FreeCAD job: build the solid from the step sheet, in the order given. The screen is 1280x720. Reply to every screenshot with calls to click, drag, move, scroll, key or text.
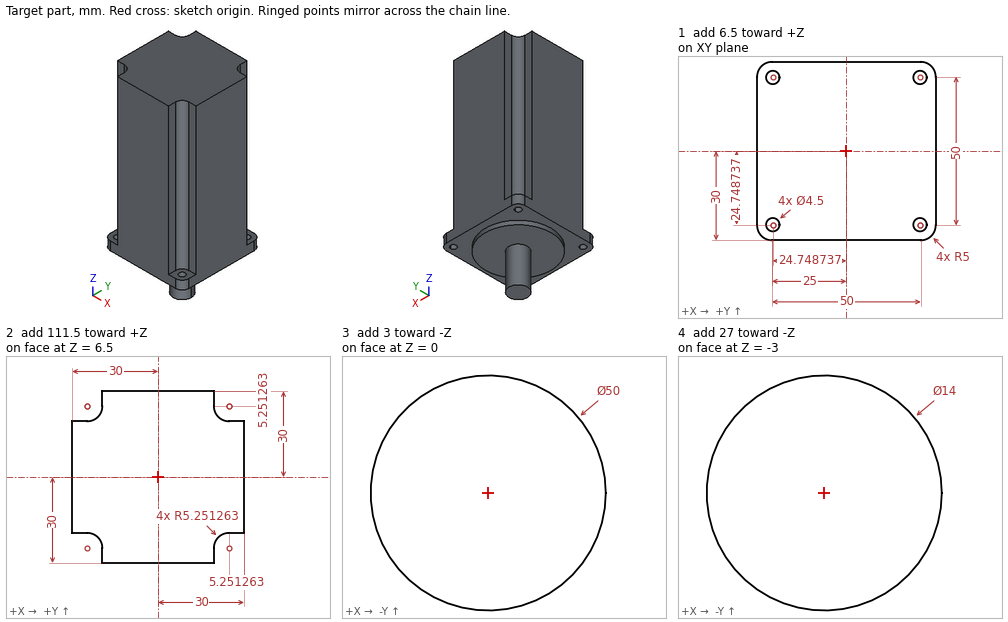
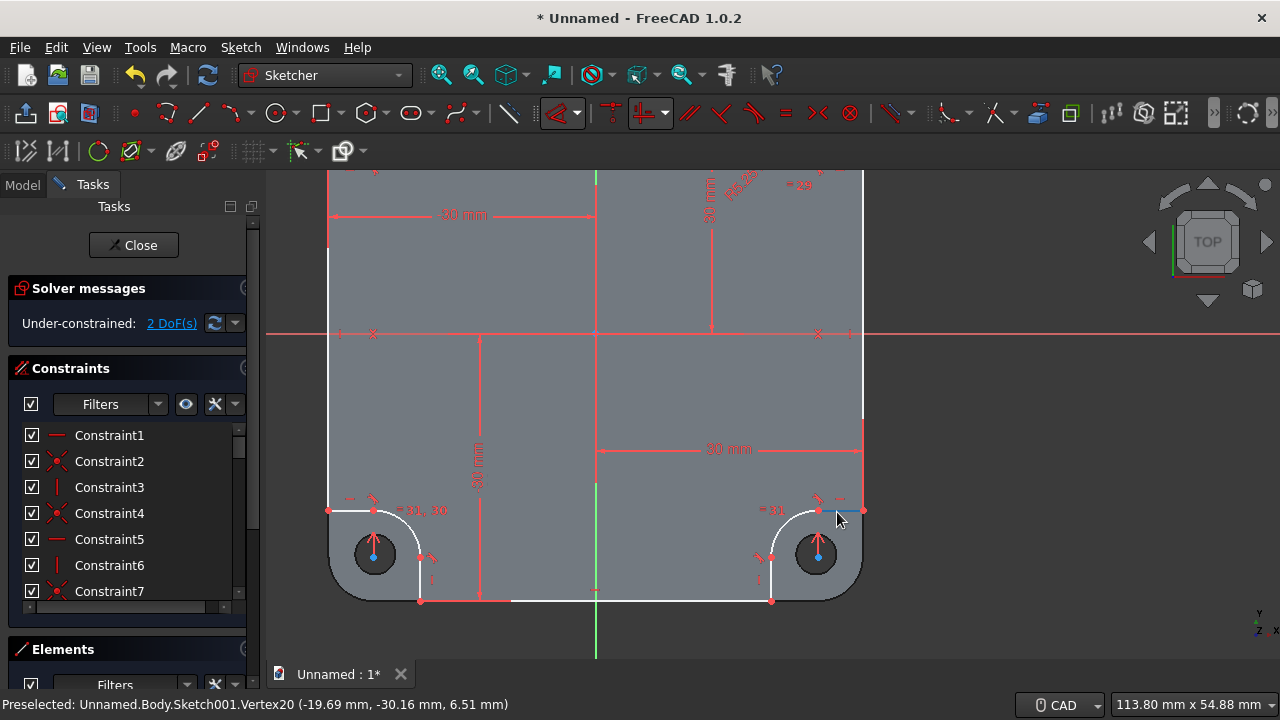
click(836, 511)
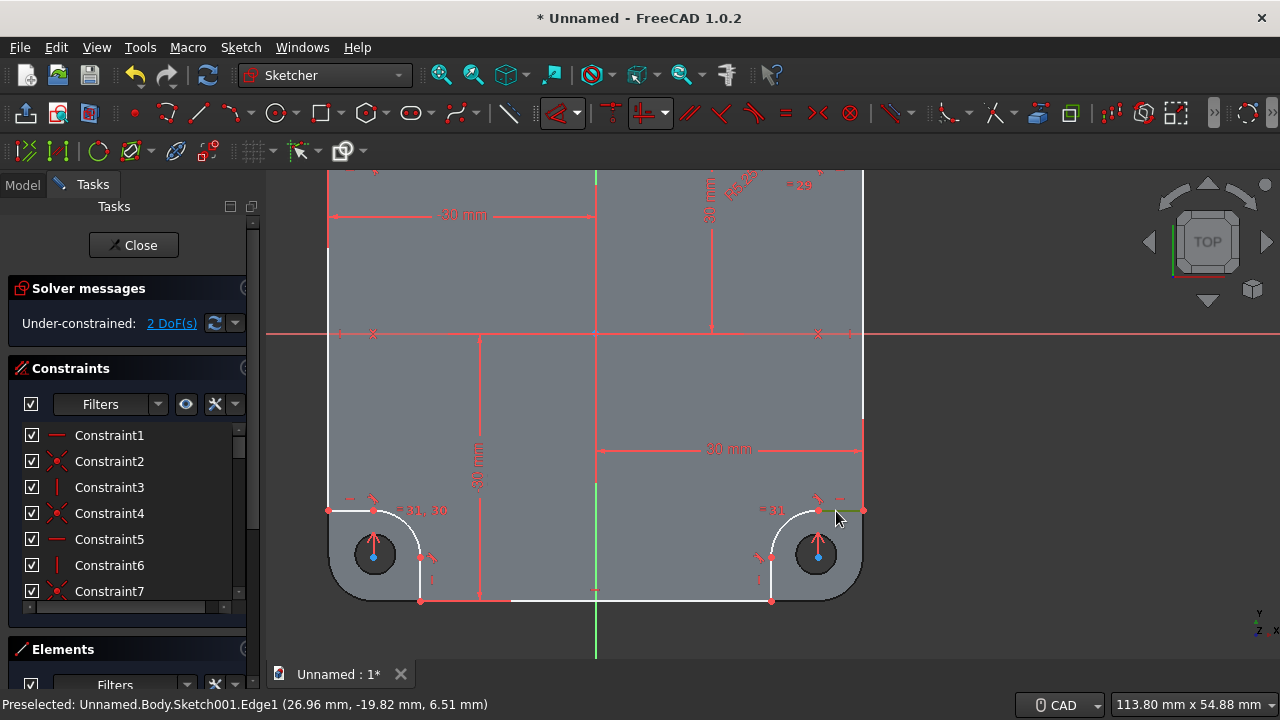
key(l)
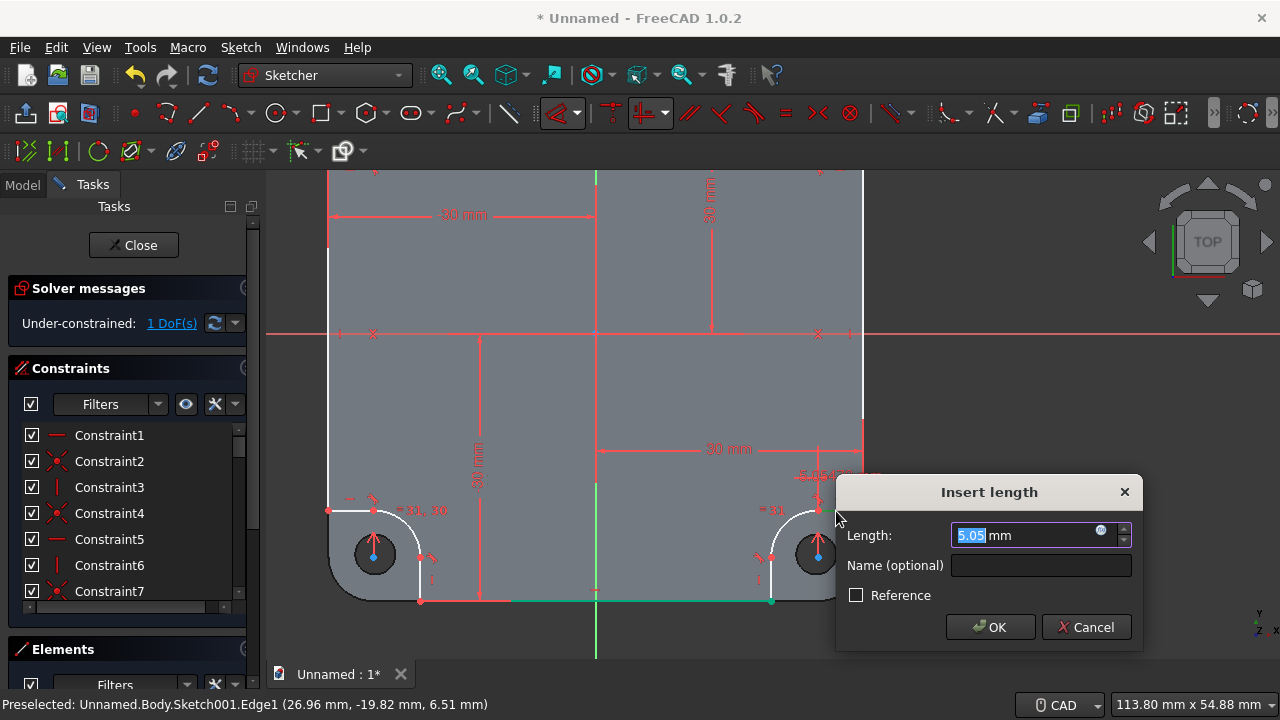
text(5.251263)
key(Return)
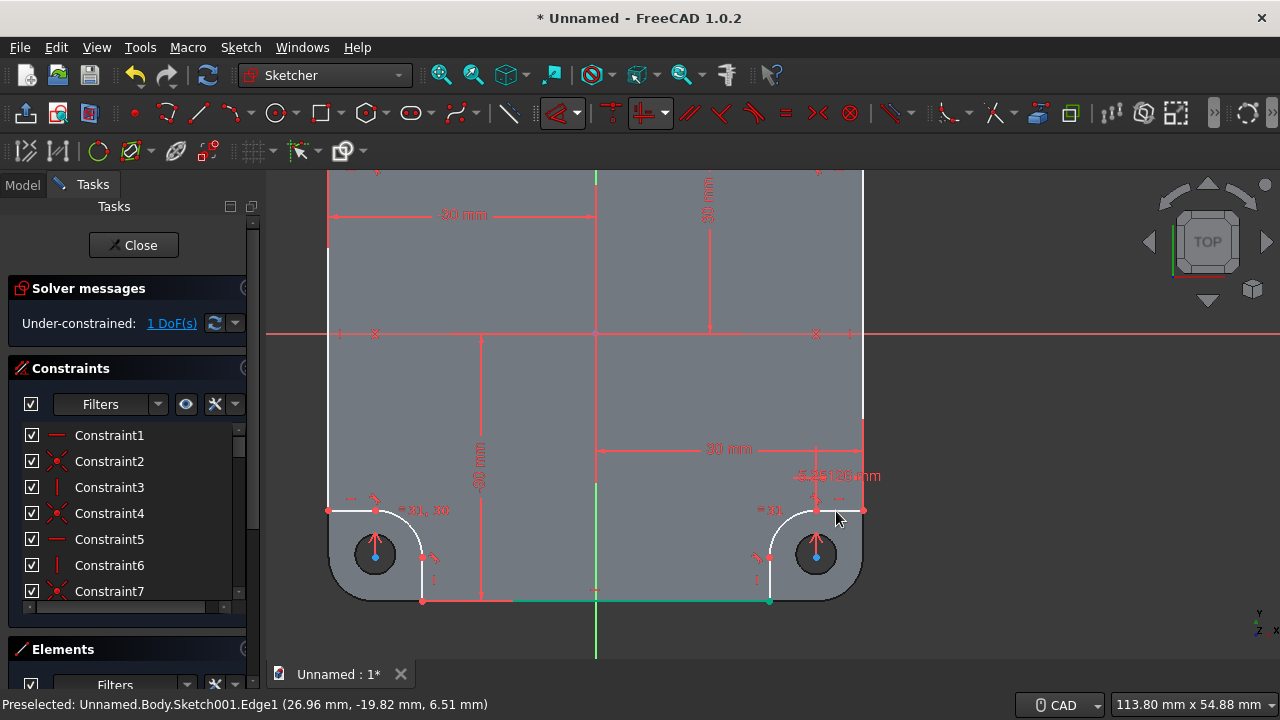
scroll(837, 512, down, 3)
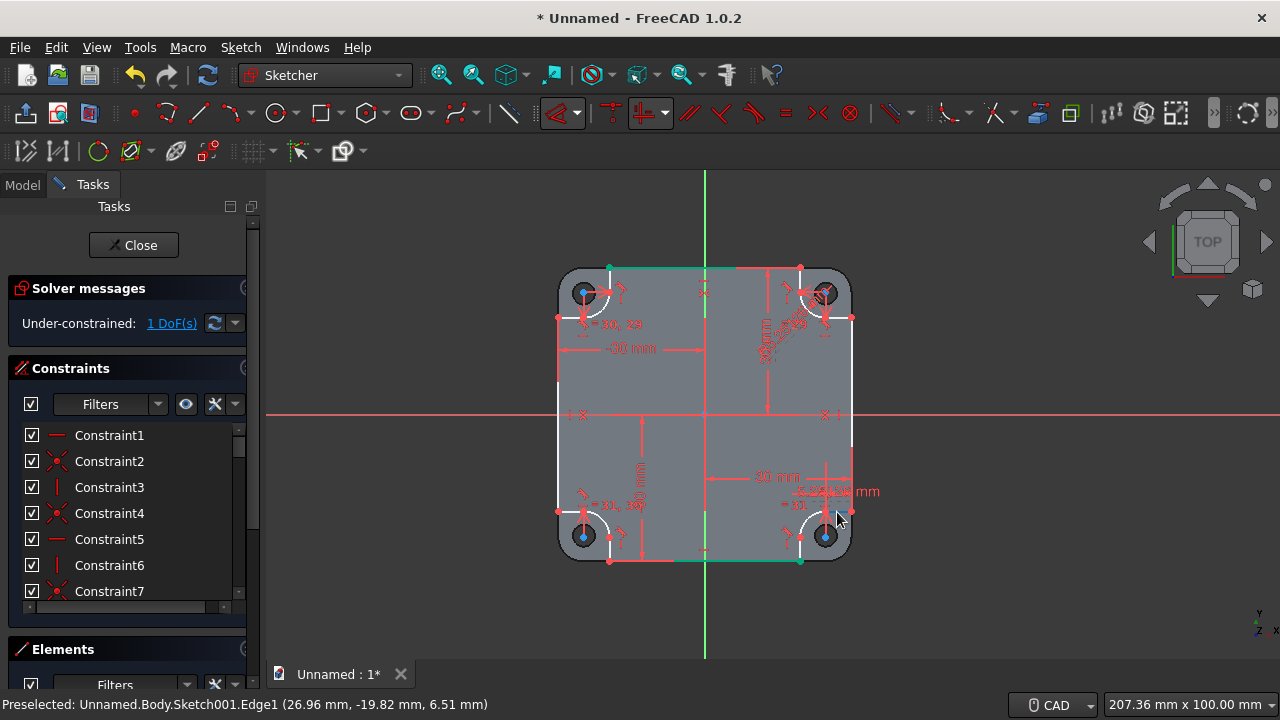
scroll(800, 285, up, 4)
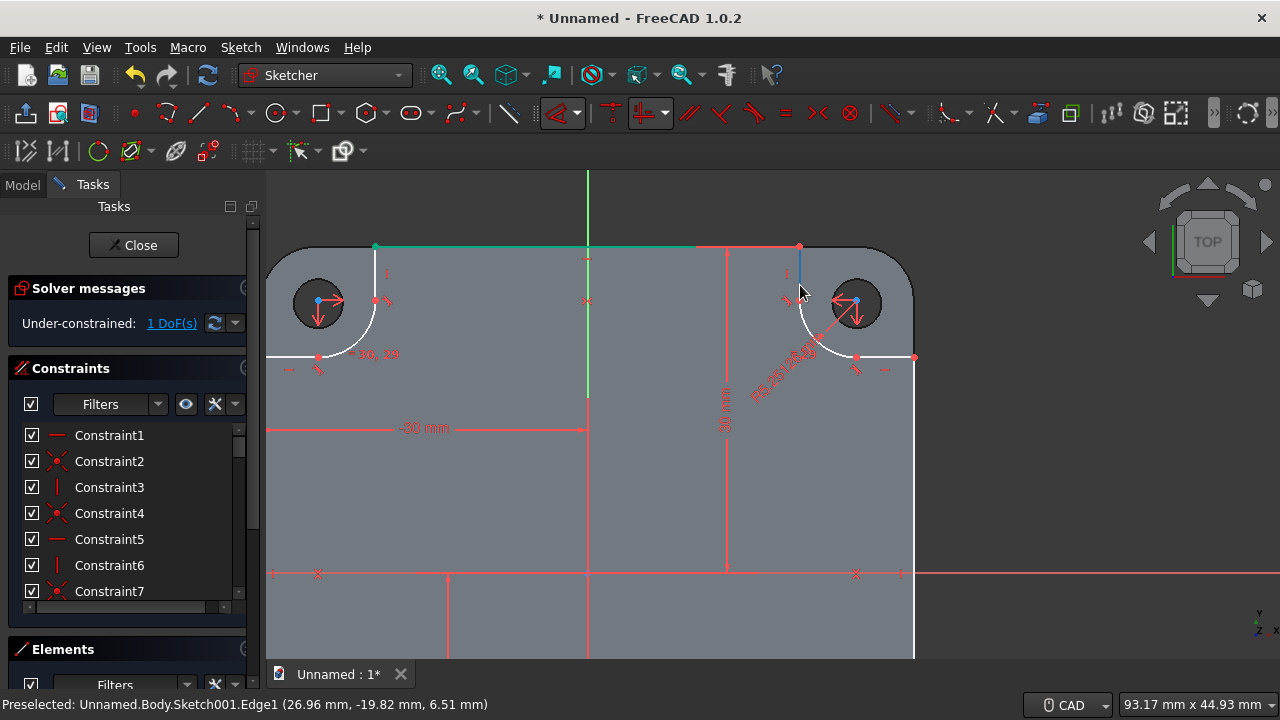
click(800, 284)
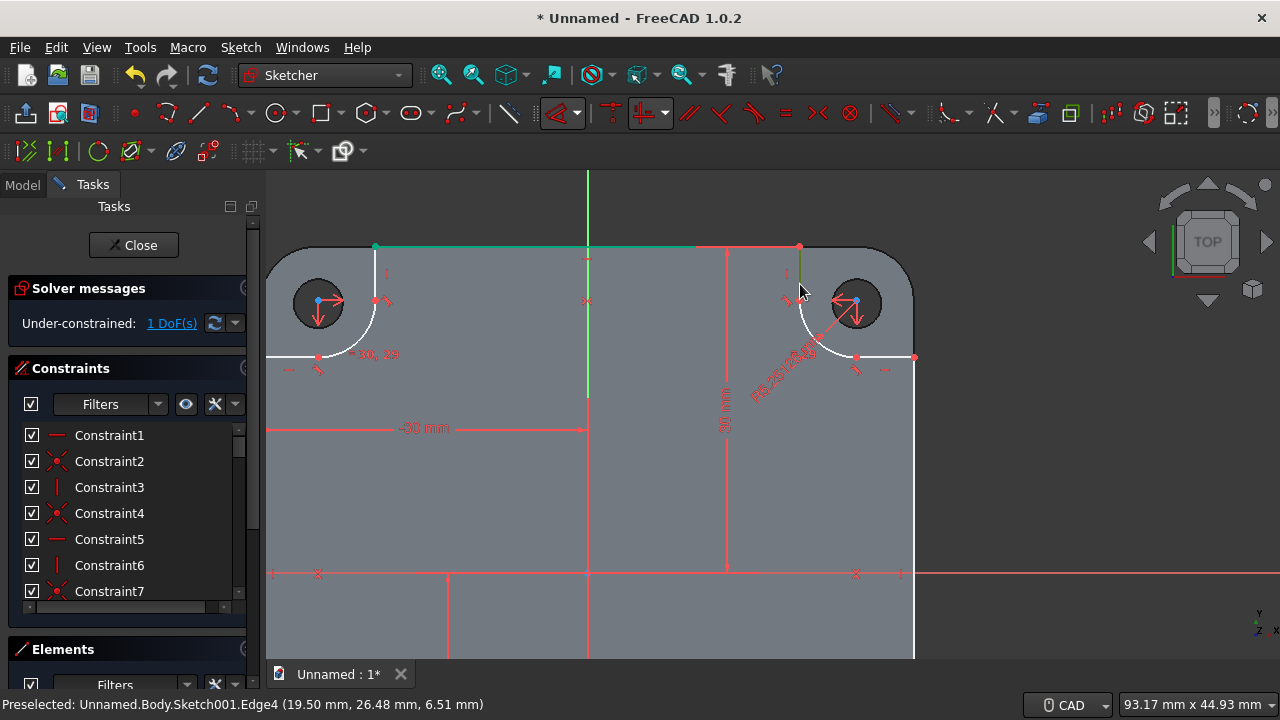
key(i)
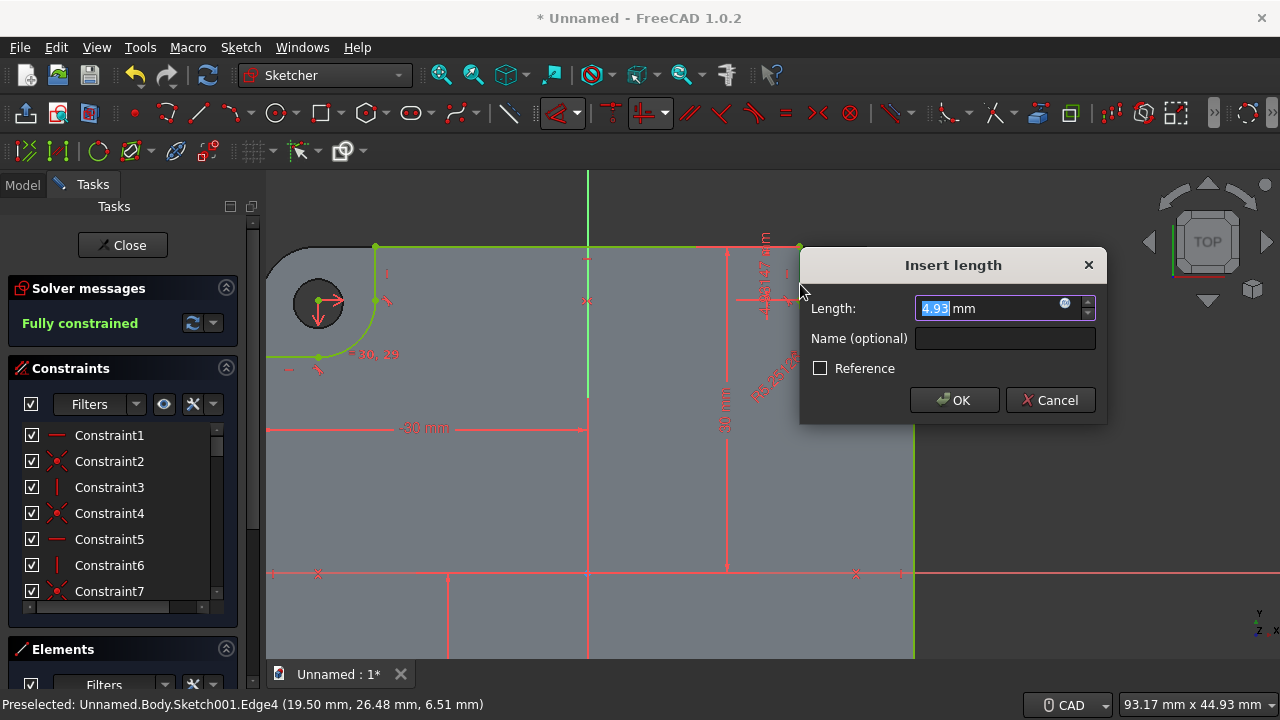
text(5.251263)
key(Return)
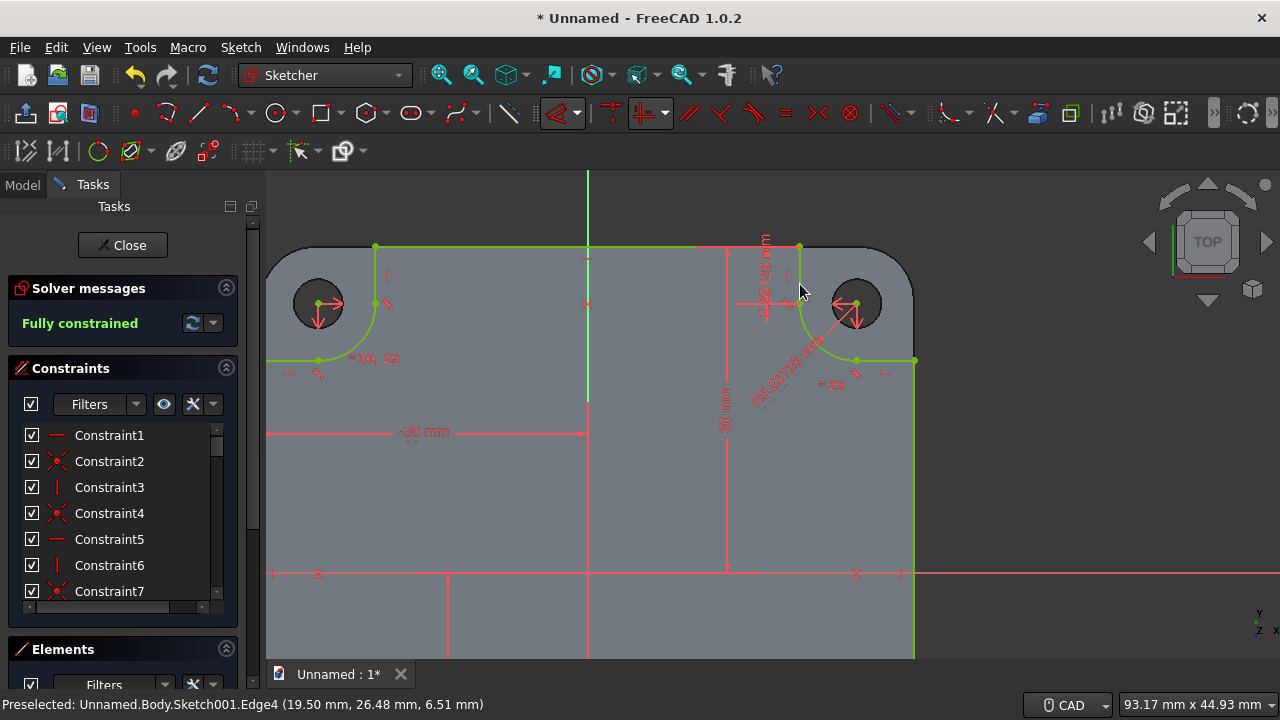
click(123, 245)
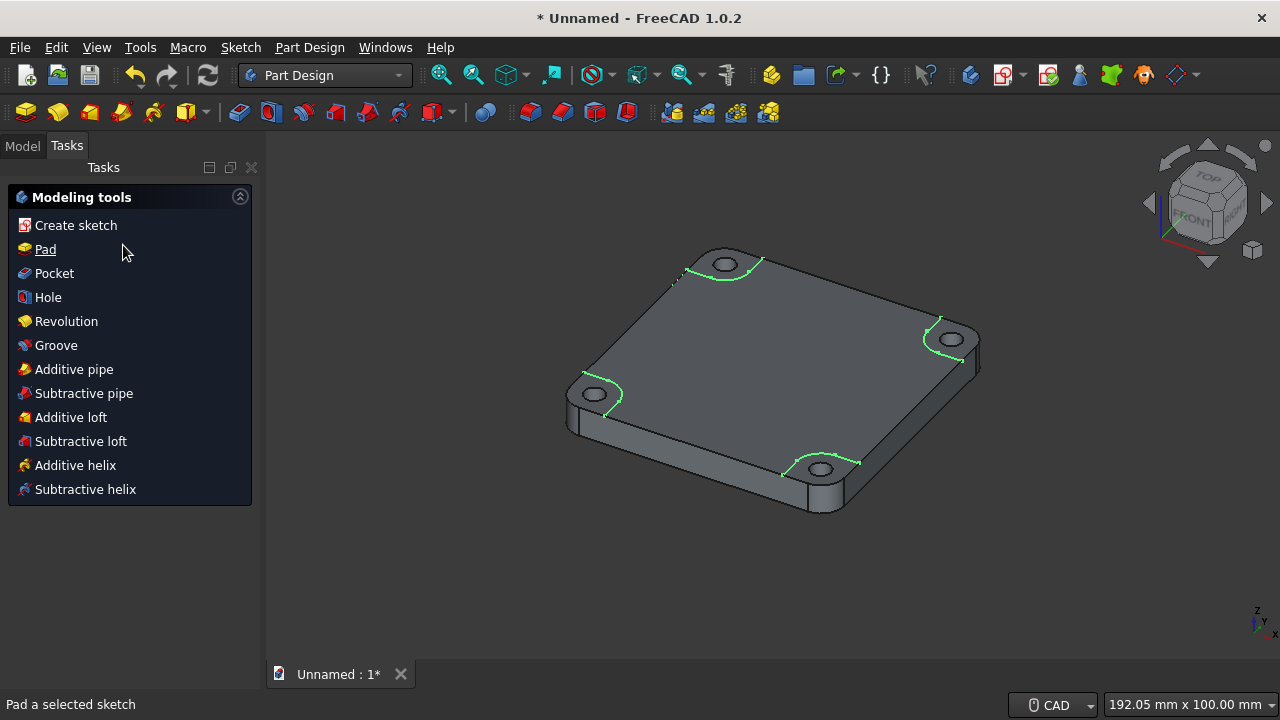
click(26, 112)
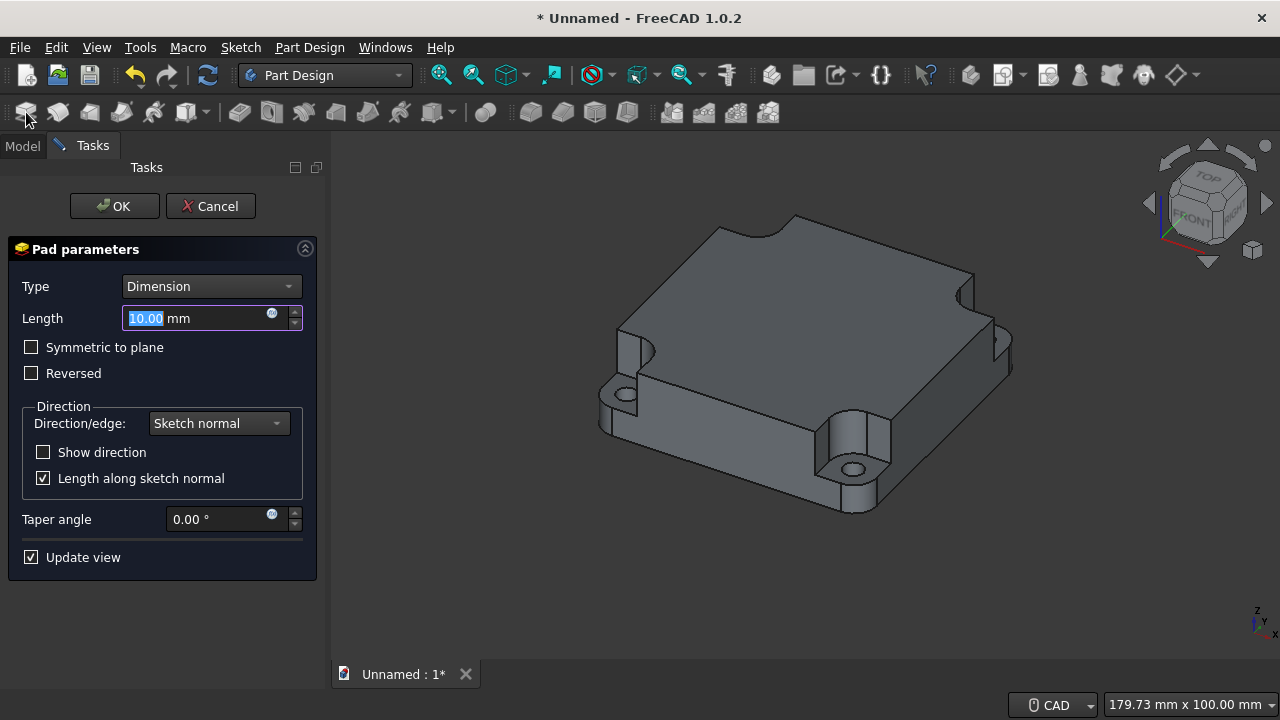
text(111.5)
key(Tab)